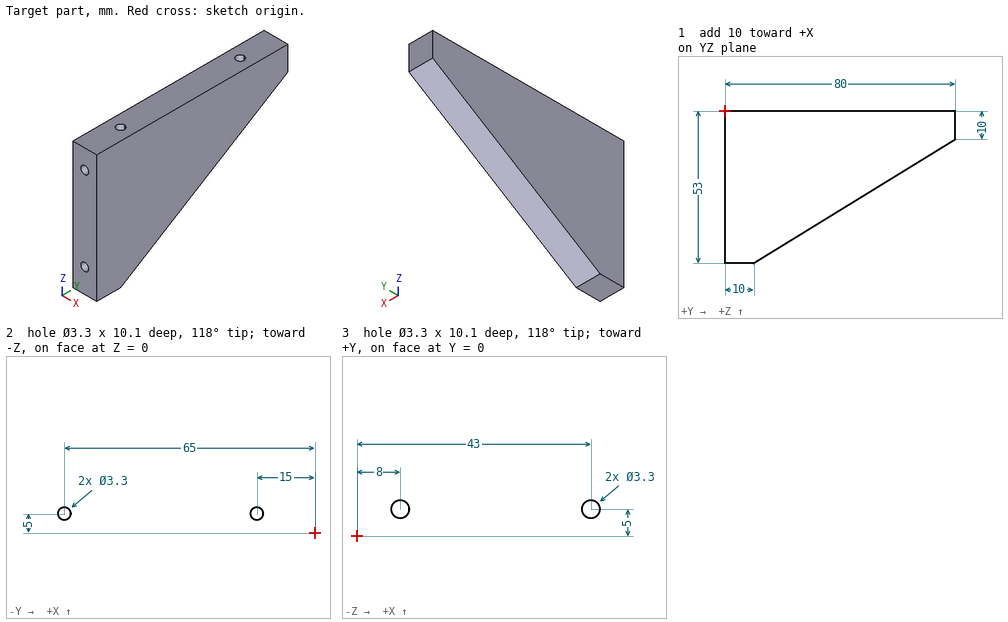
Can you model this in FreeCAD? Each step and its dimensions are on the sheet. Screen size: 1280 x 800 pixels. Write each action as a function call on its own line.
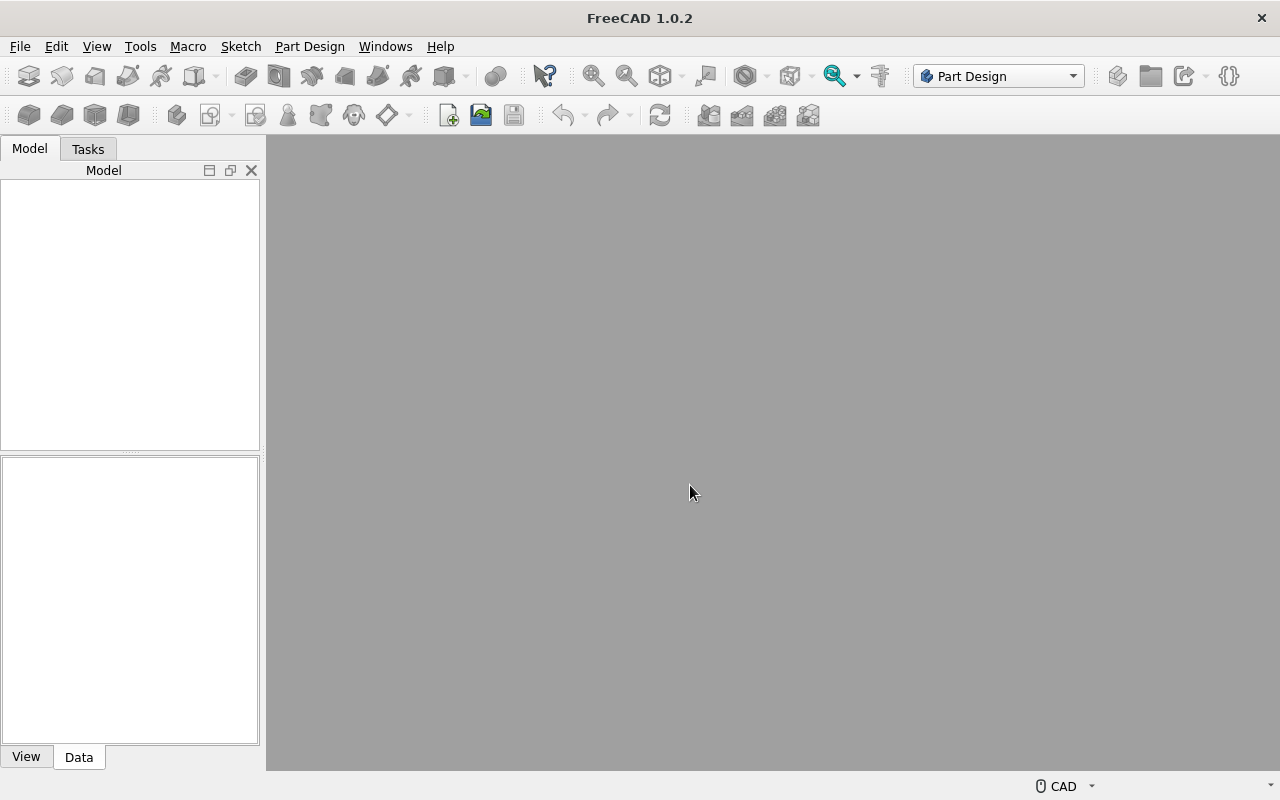
key(ctrl+n)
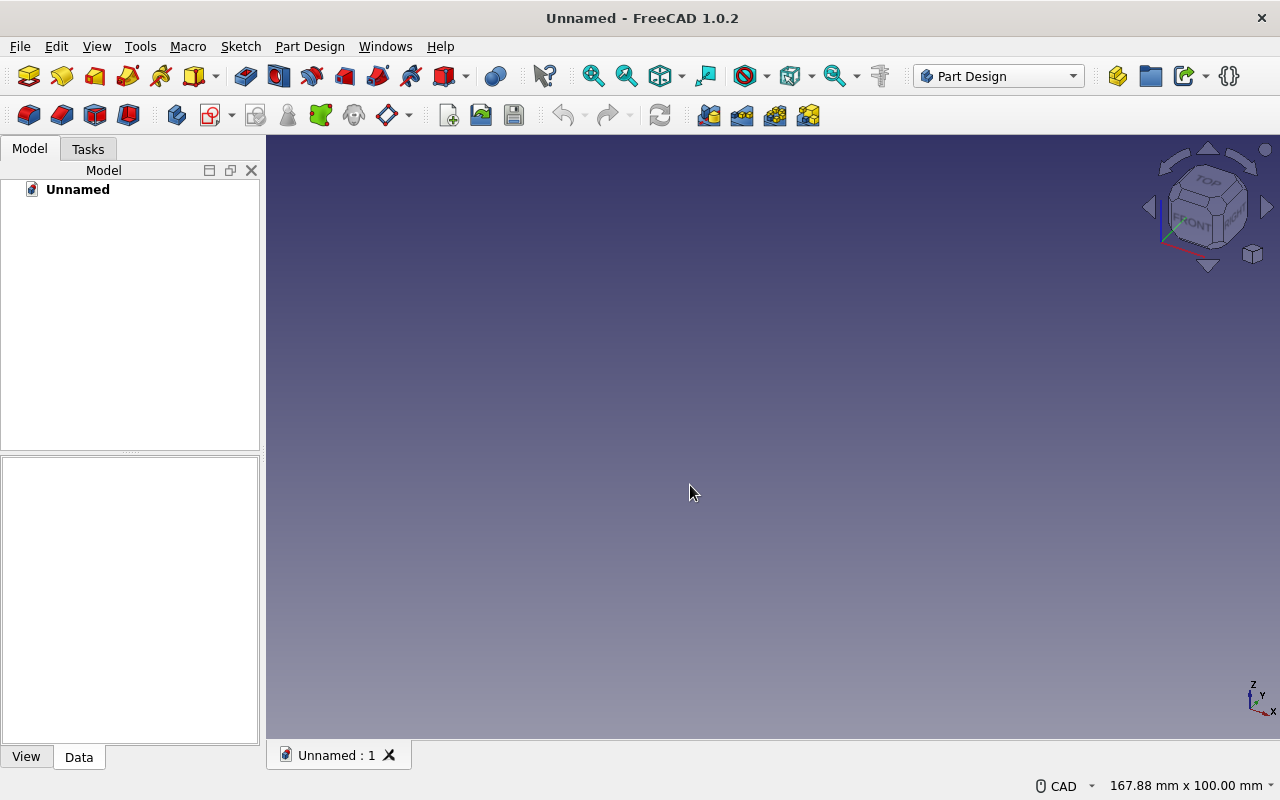
click(210, 116)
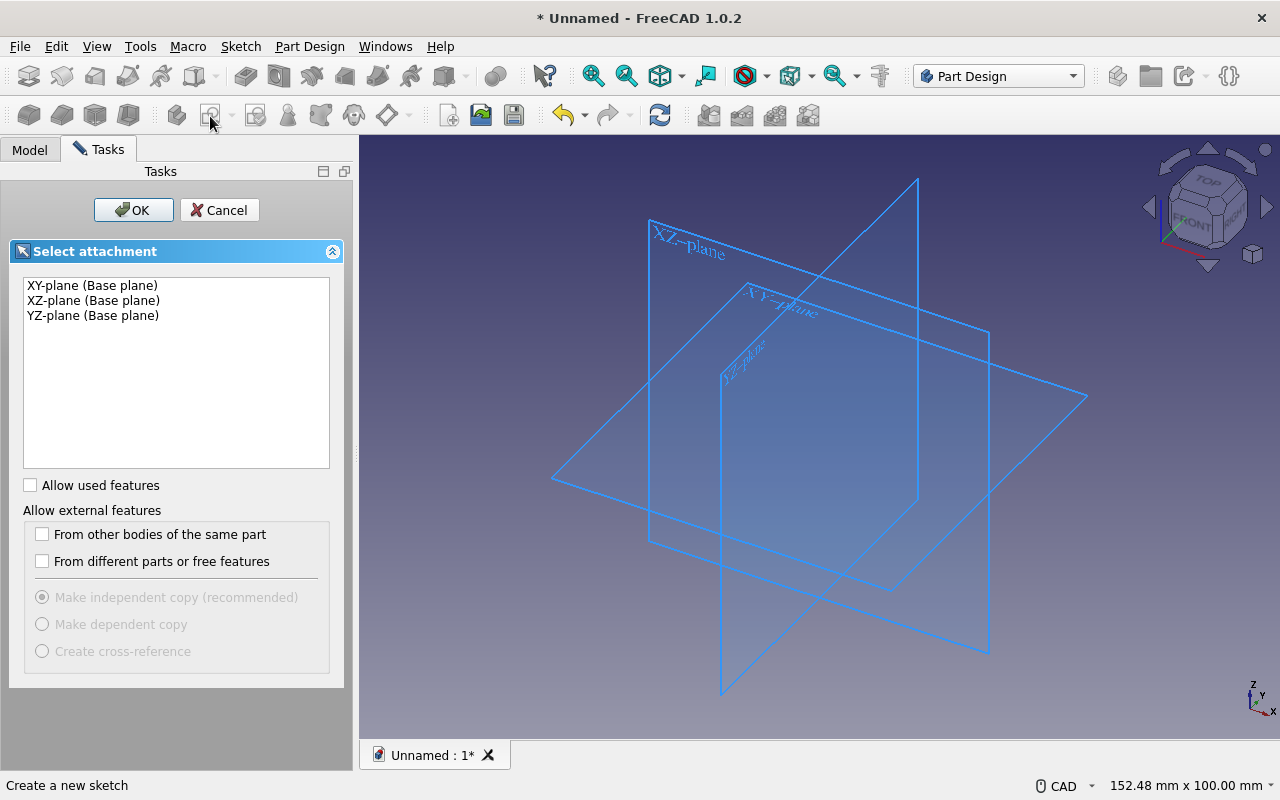
click(84, 316)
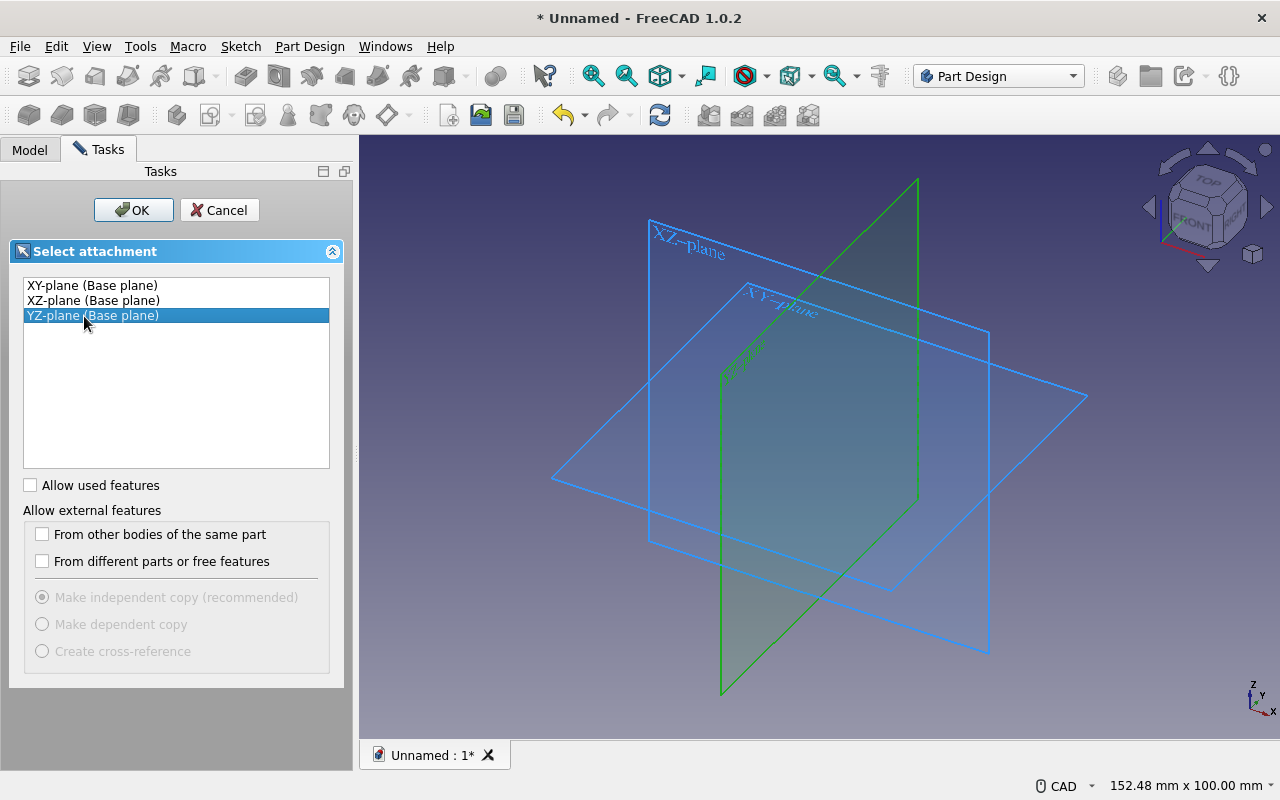
click(134, 210)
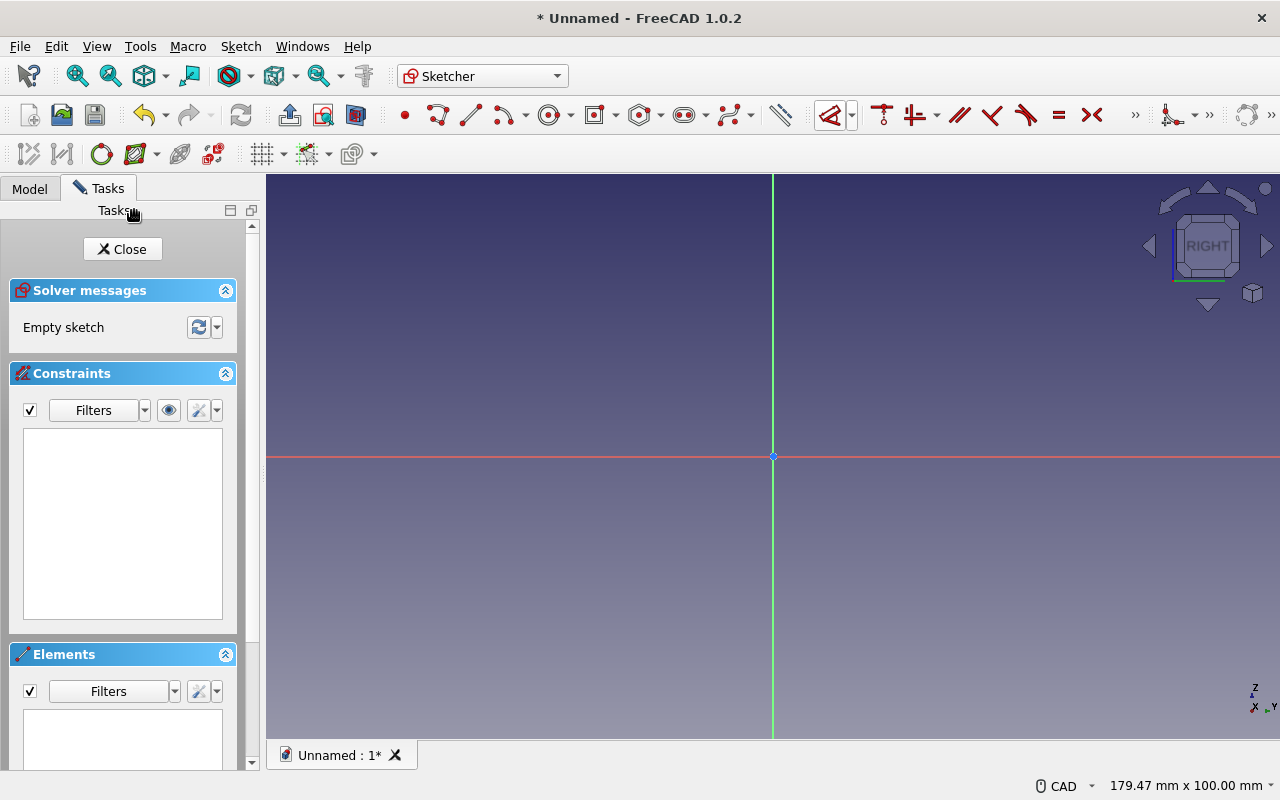
scroll(294, 202, down, 1)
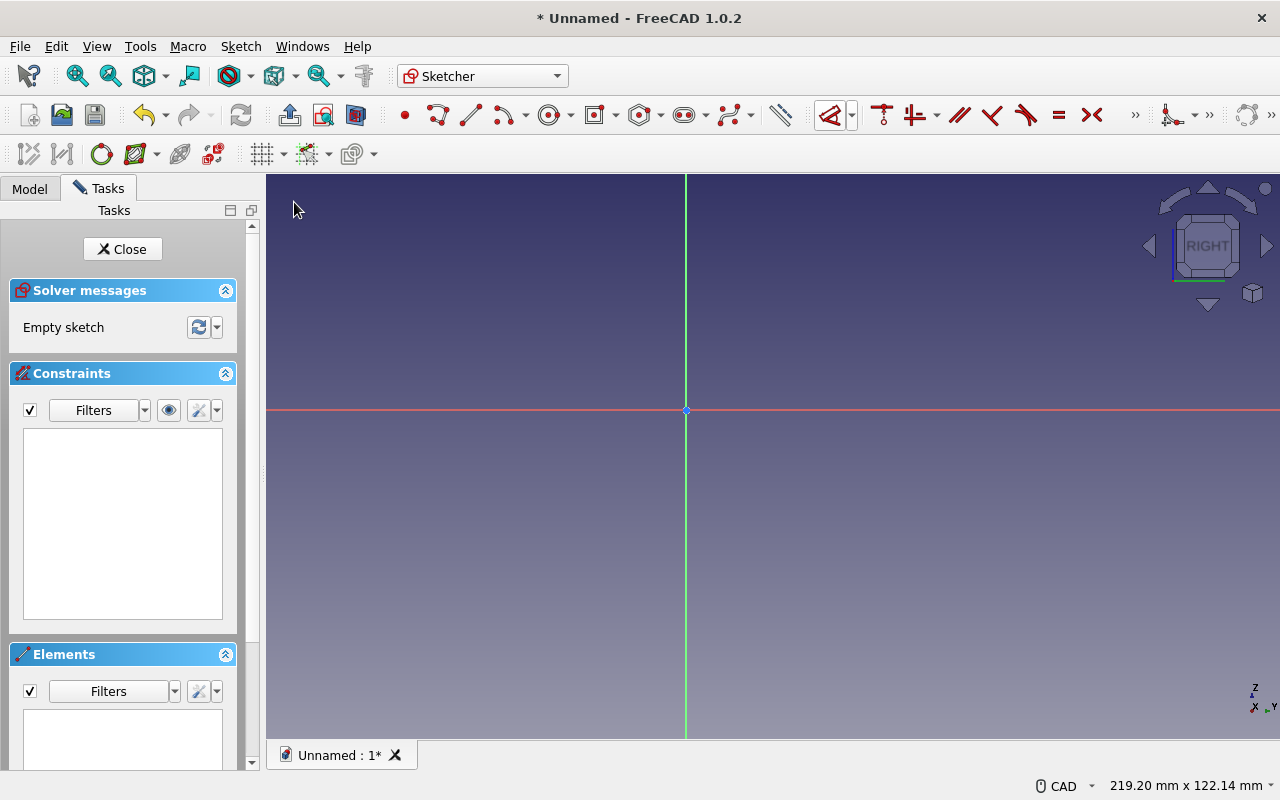
scroll(1115, 688, up, 2)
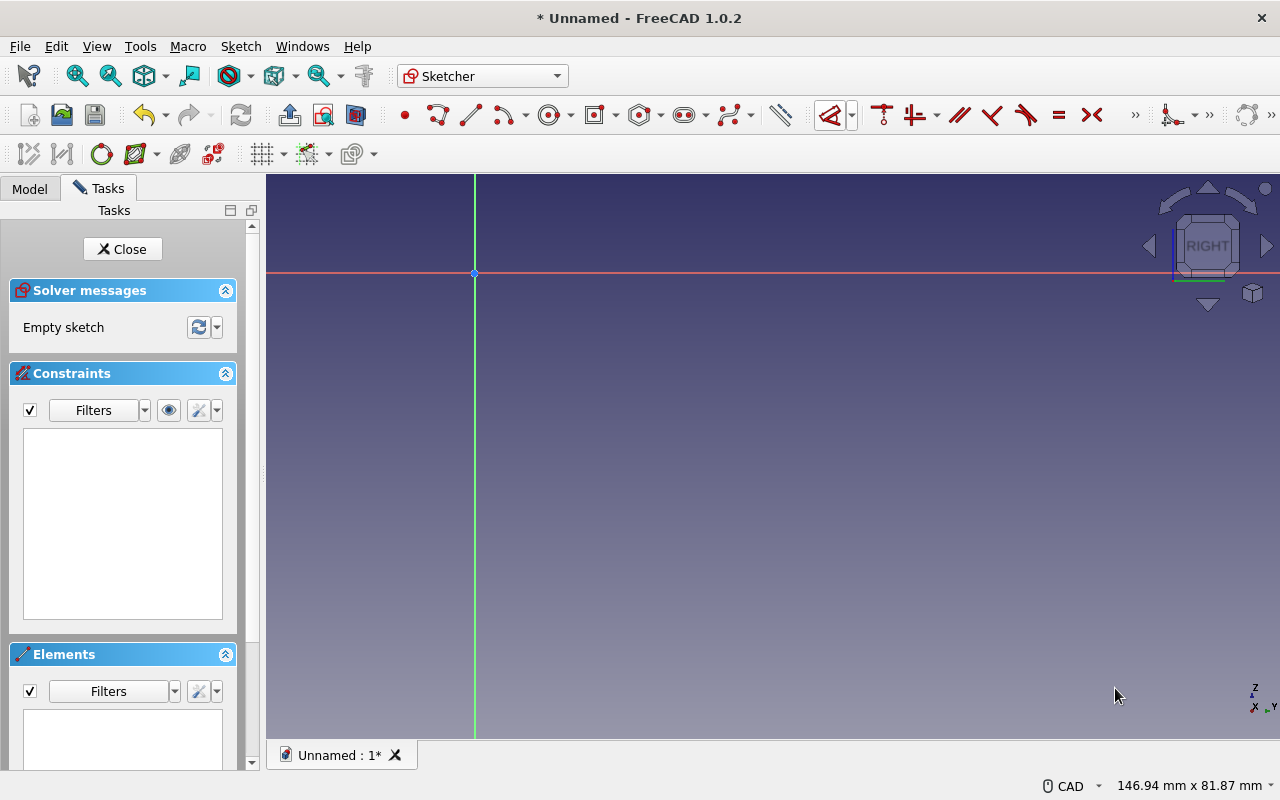
click(438, 116)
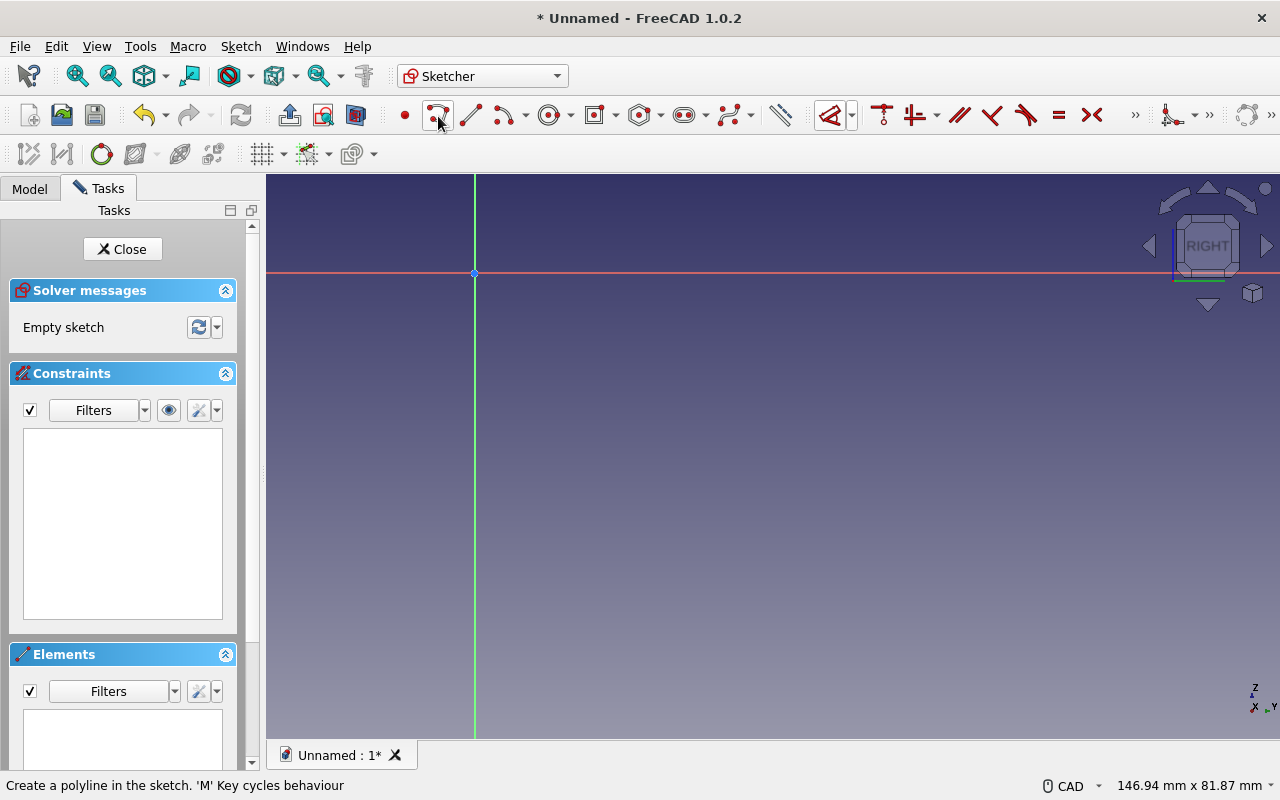
click(475, 273)
click(484, 639)
click(544, 639)
click(1027, 342)
click(1027, 282)
click(475, 273)
key(Escape)
key(Escape)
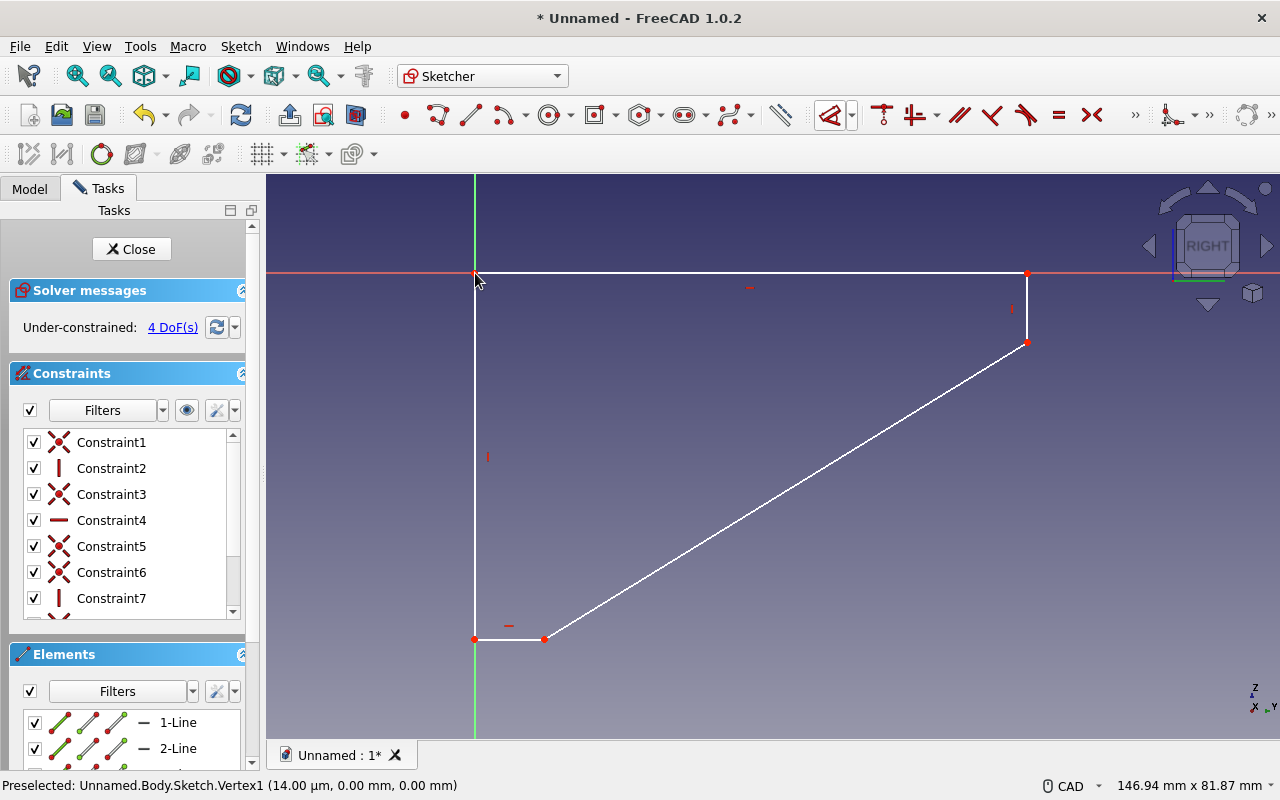
click(830, 116)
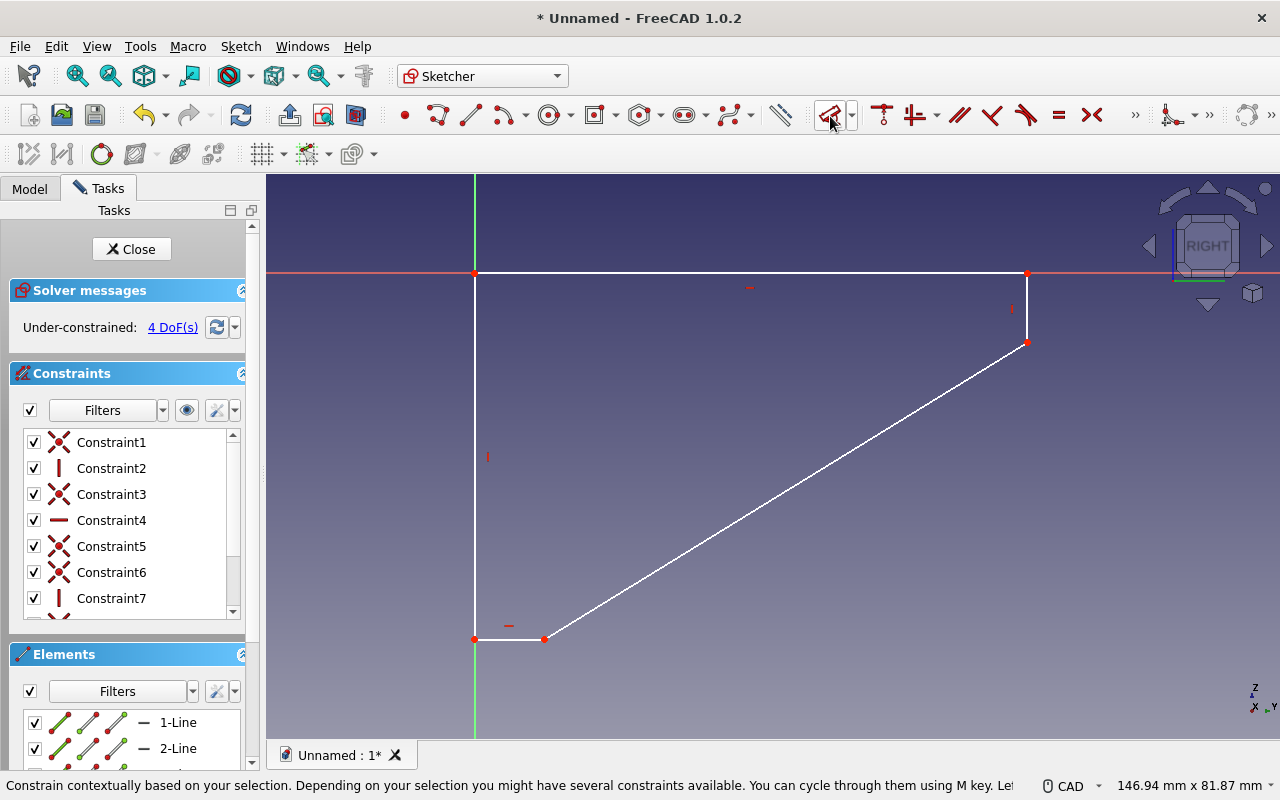
click(475, 383)
click(441, 457)